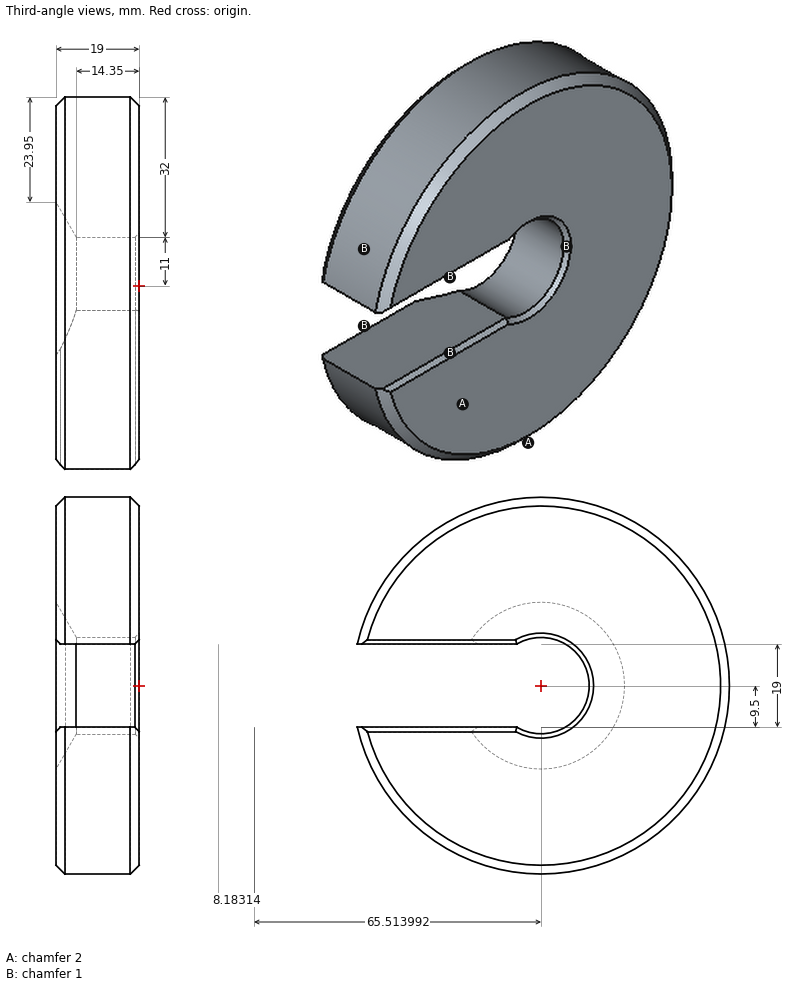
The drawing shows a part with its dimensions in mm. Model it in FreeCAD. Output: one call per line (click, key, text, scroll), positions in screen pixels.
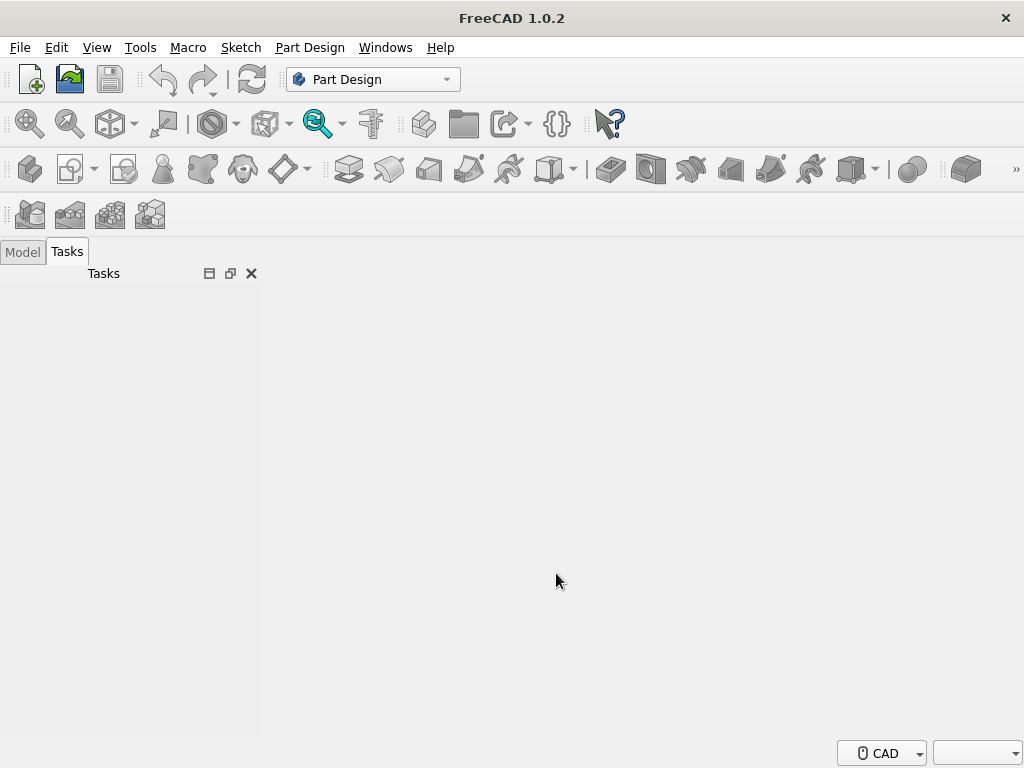
click(30, 80)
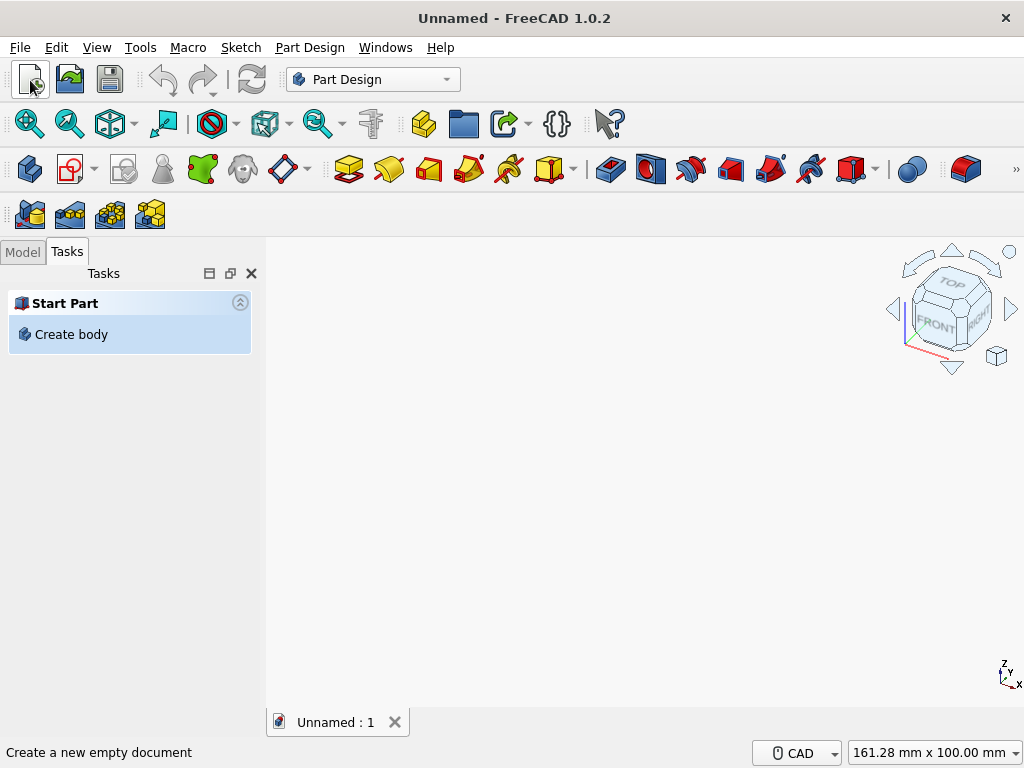
click(70, 170)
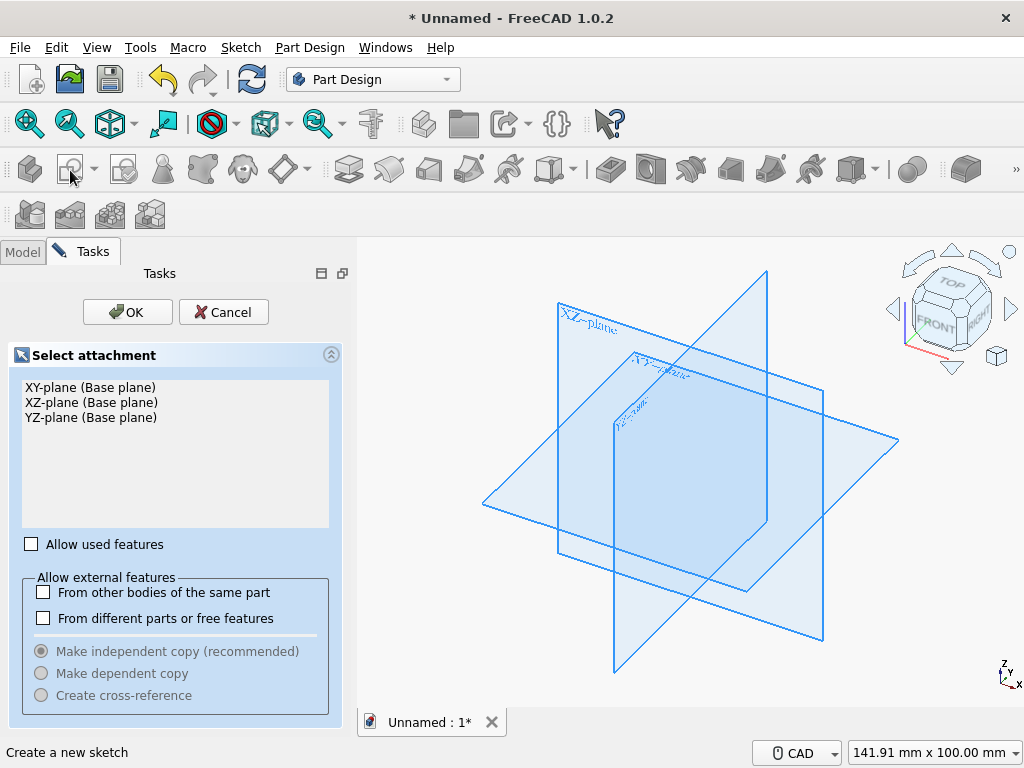
click(82, 388)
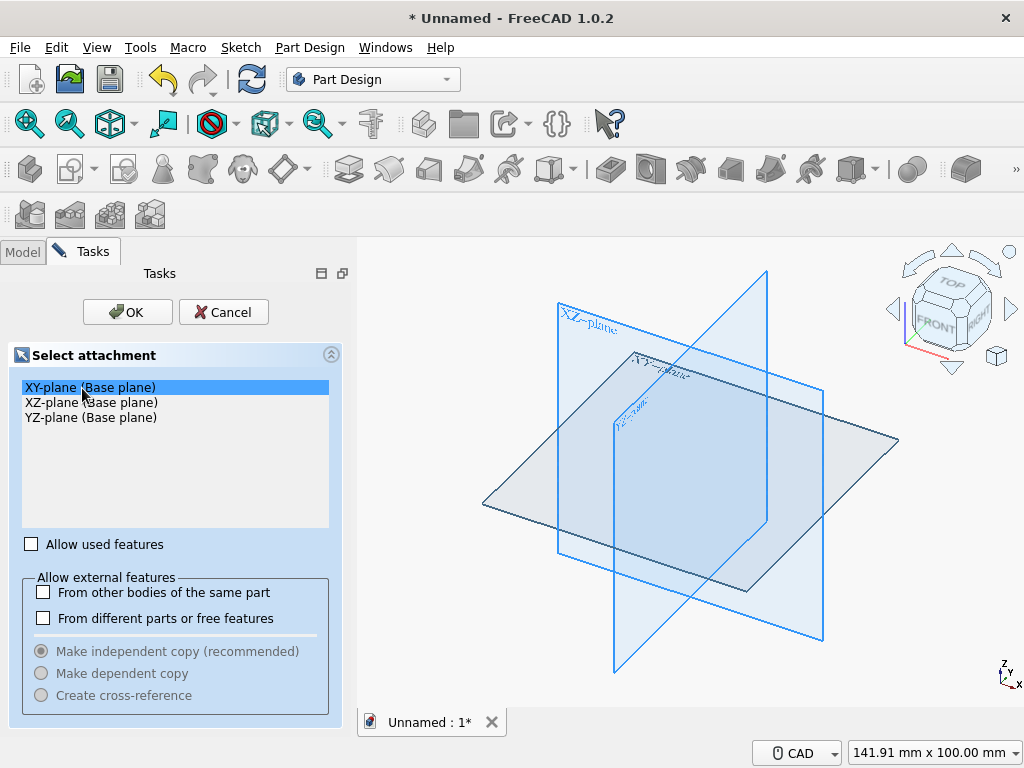
click(128, 312)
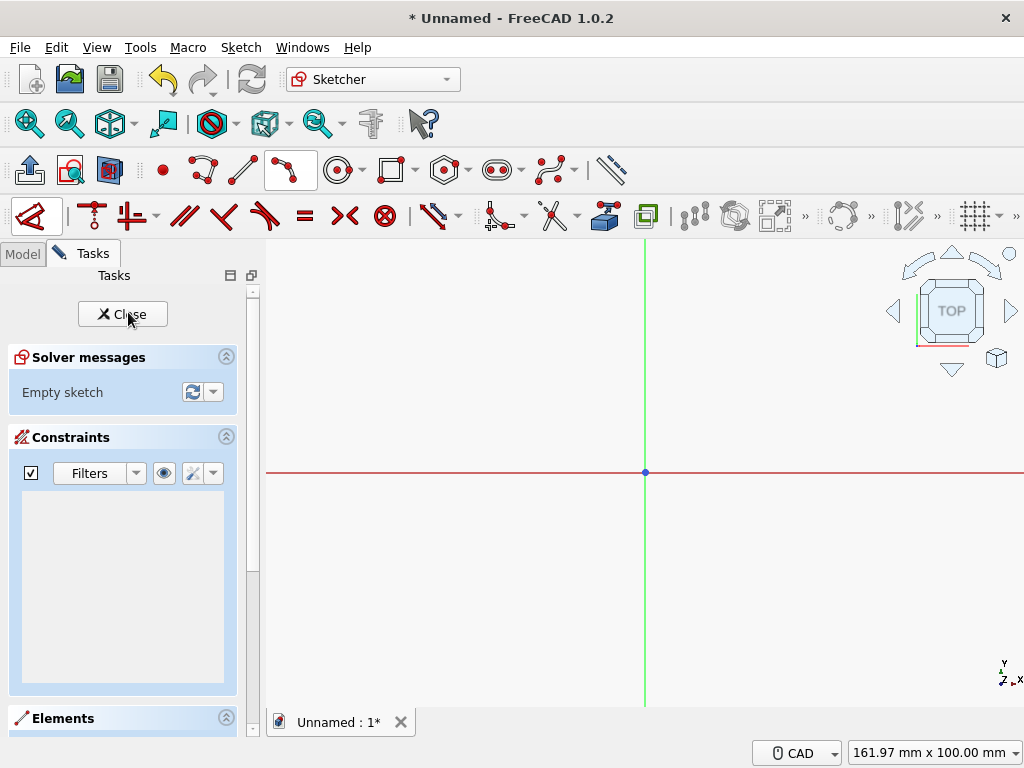
scroll(468, 679, down, 1)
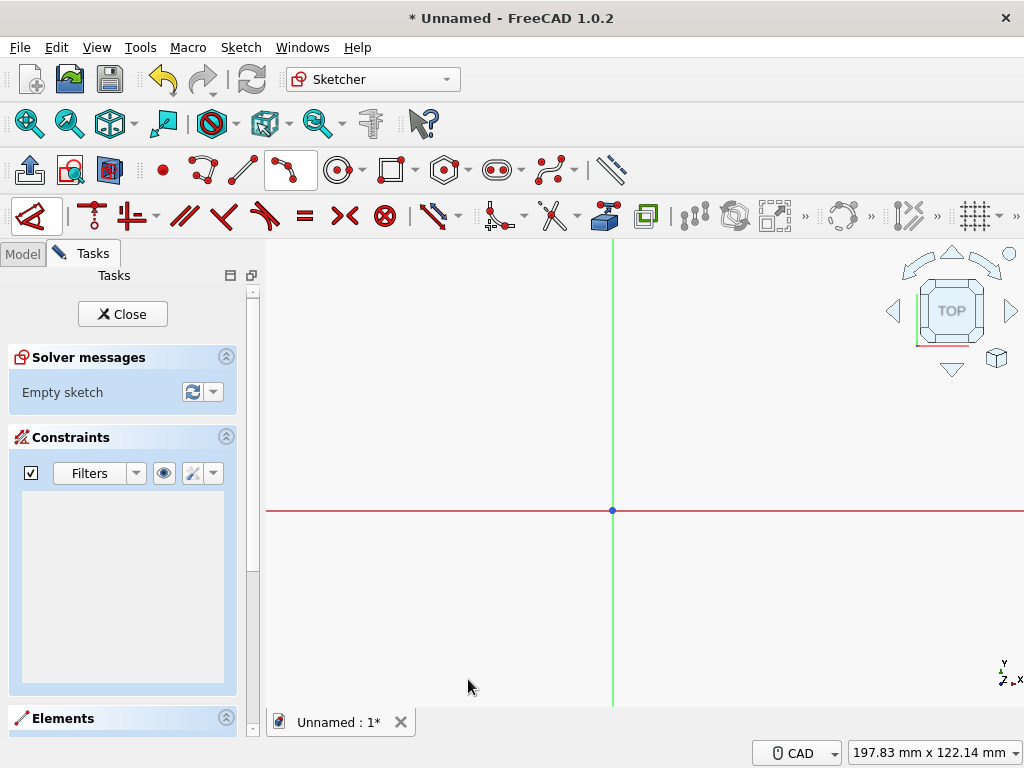
scroll(577, 374, up, 3)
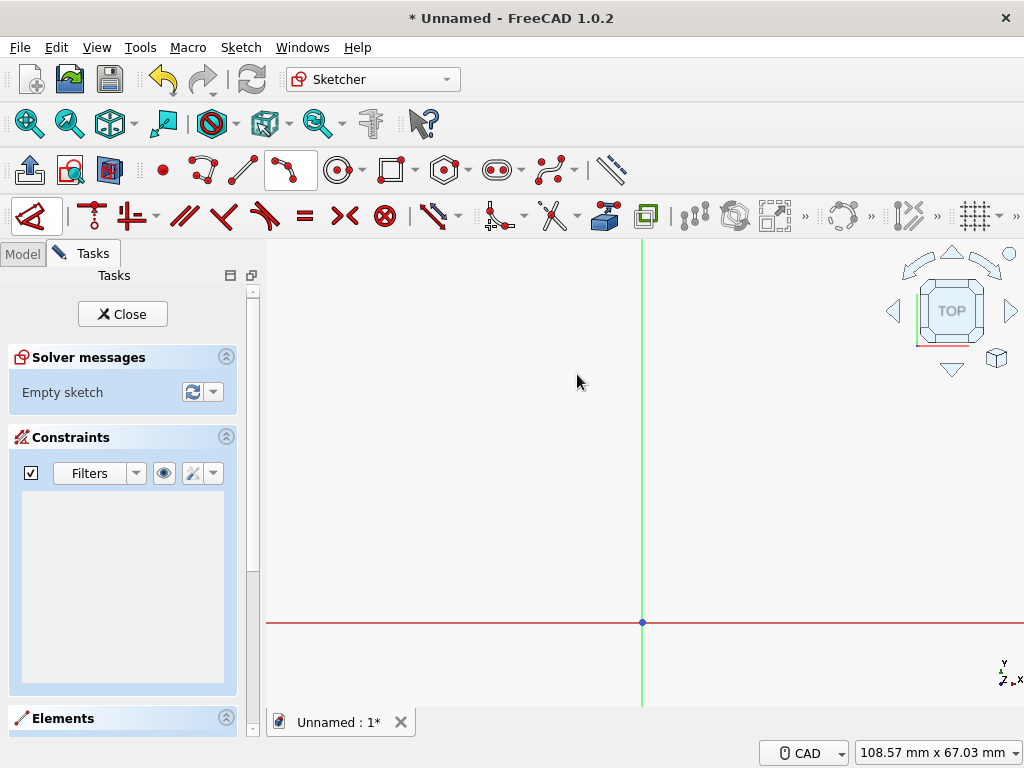
key(g)
key(m)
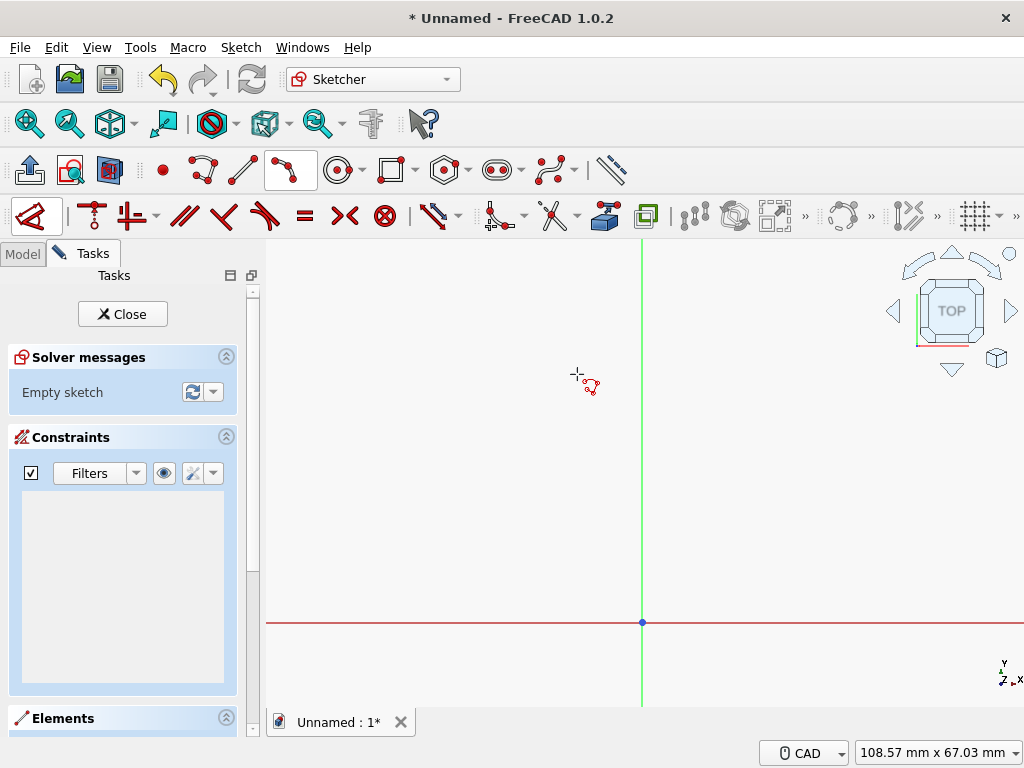
click(642, 546)
click(633, 322)
click(510, 322)
click(510, 490)
click(542, 546)
click(642, 547)
key(Escape)
key(Escape)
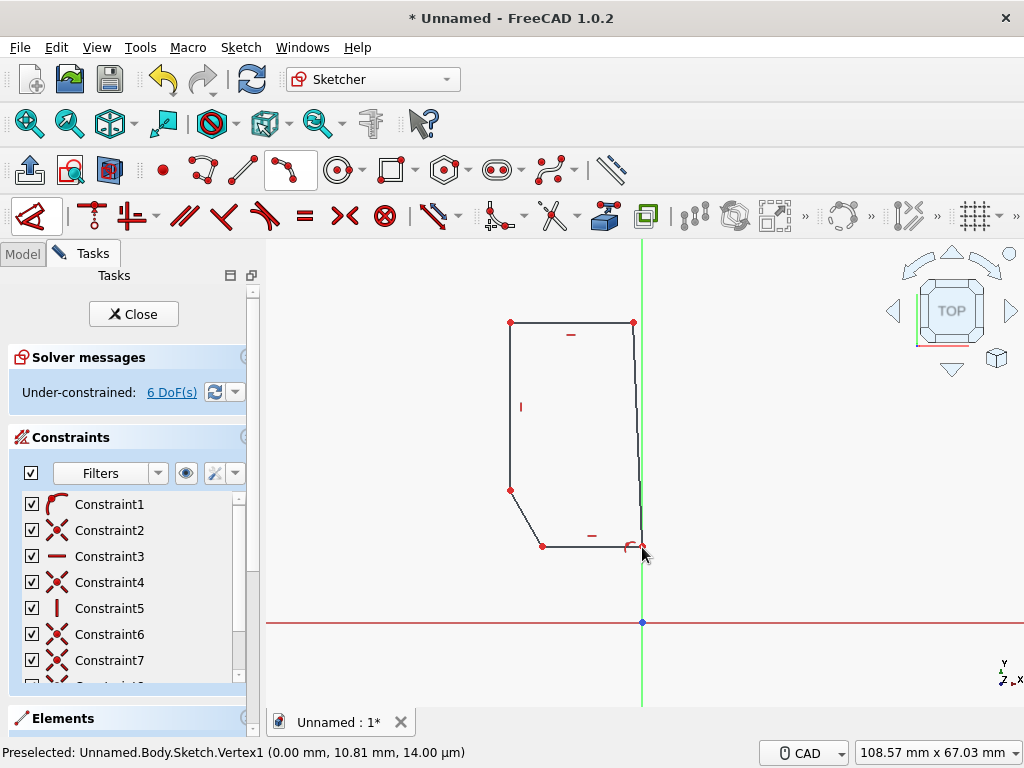
click(639, 480)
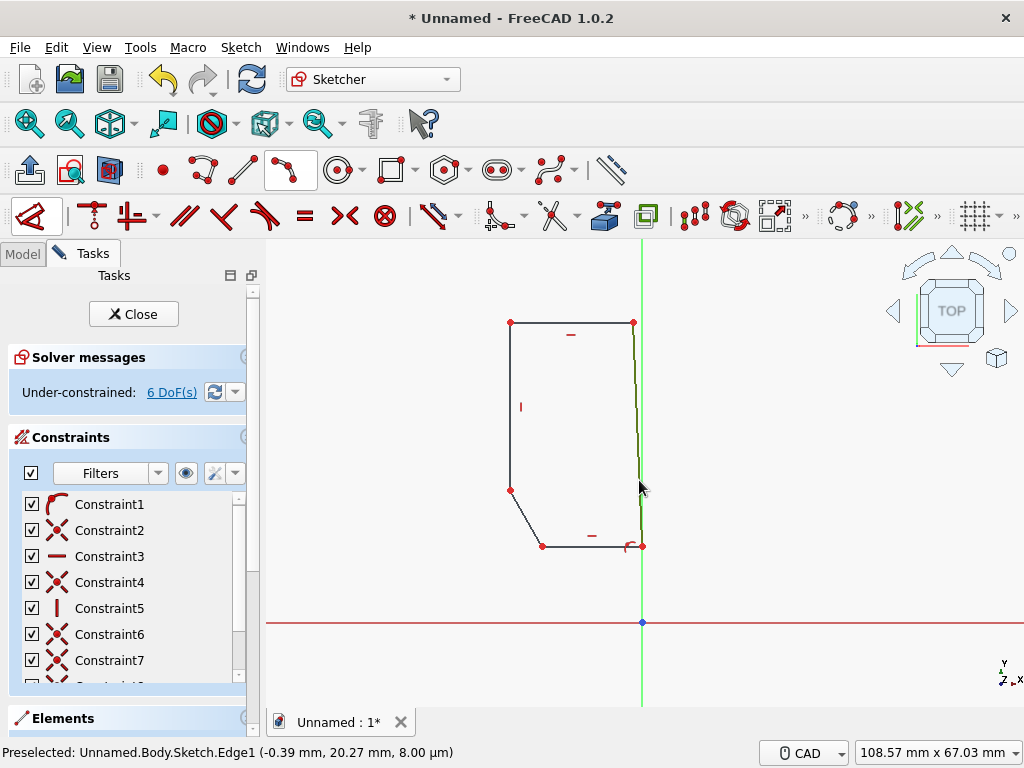
key(v)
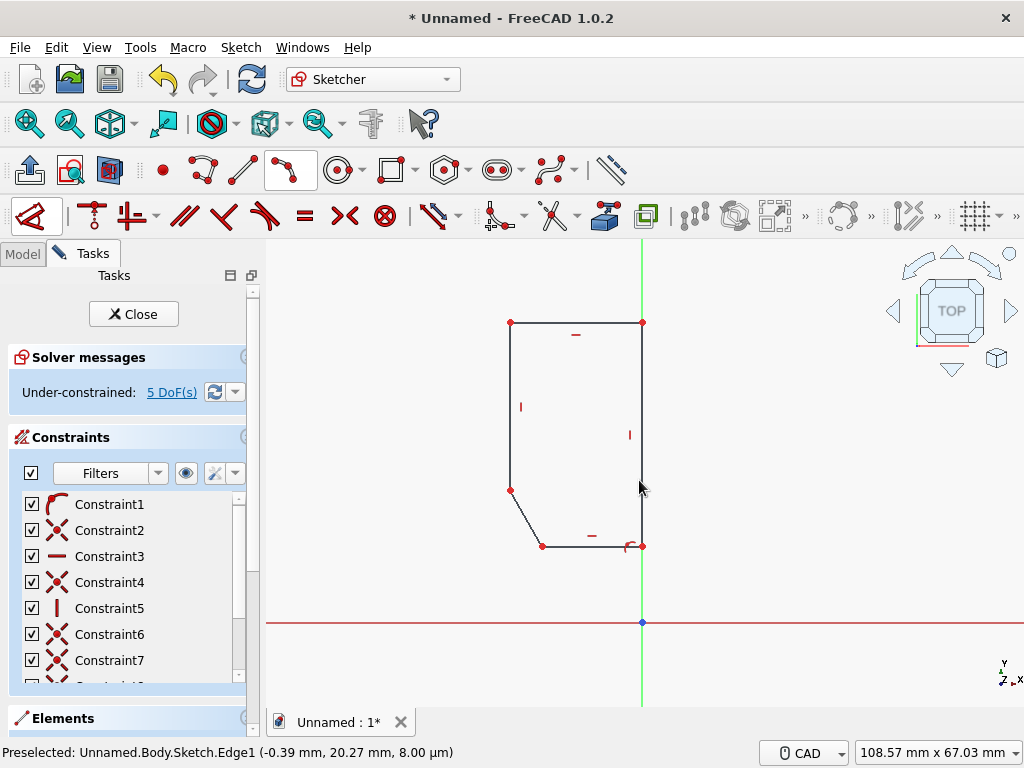
click(642, 480)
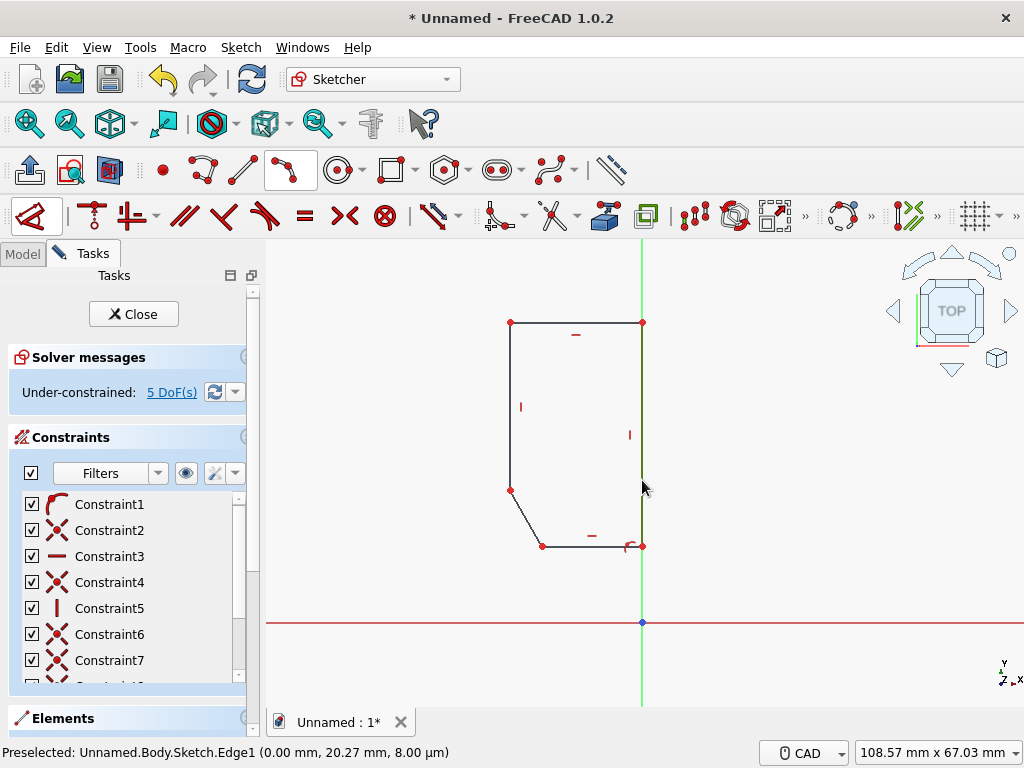
key(i)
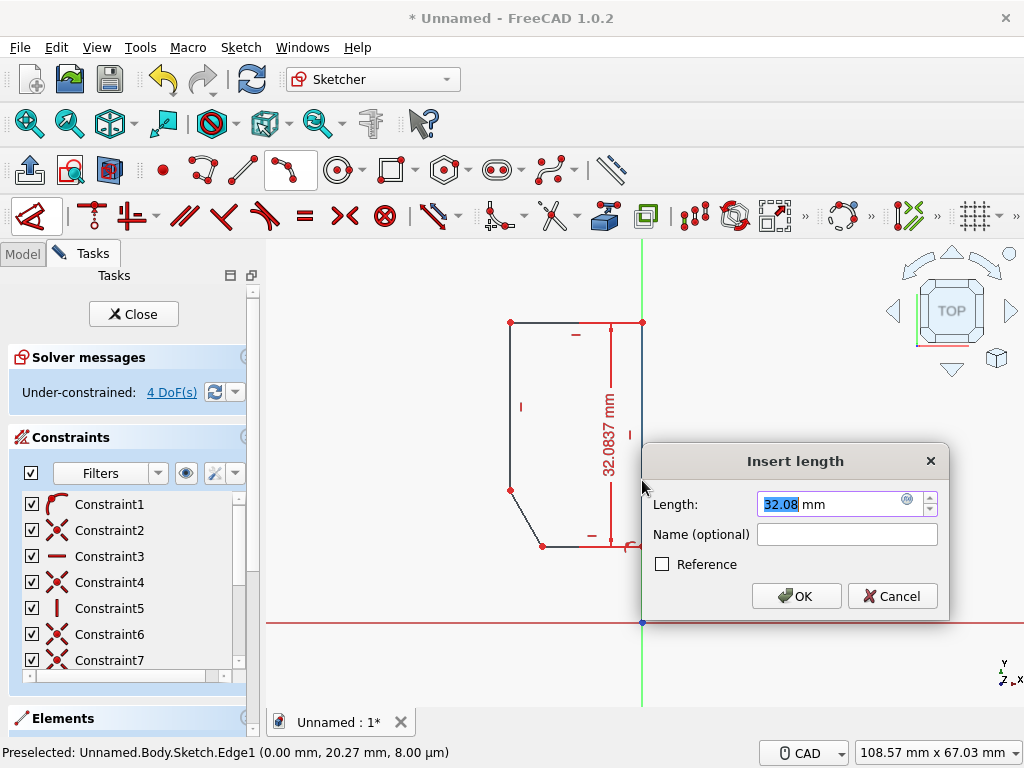
text(32)
key(Return)